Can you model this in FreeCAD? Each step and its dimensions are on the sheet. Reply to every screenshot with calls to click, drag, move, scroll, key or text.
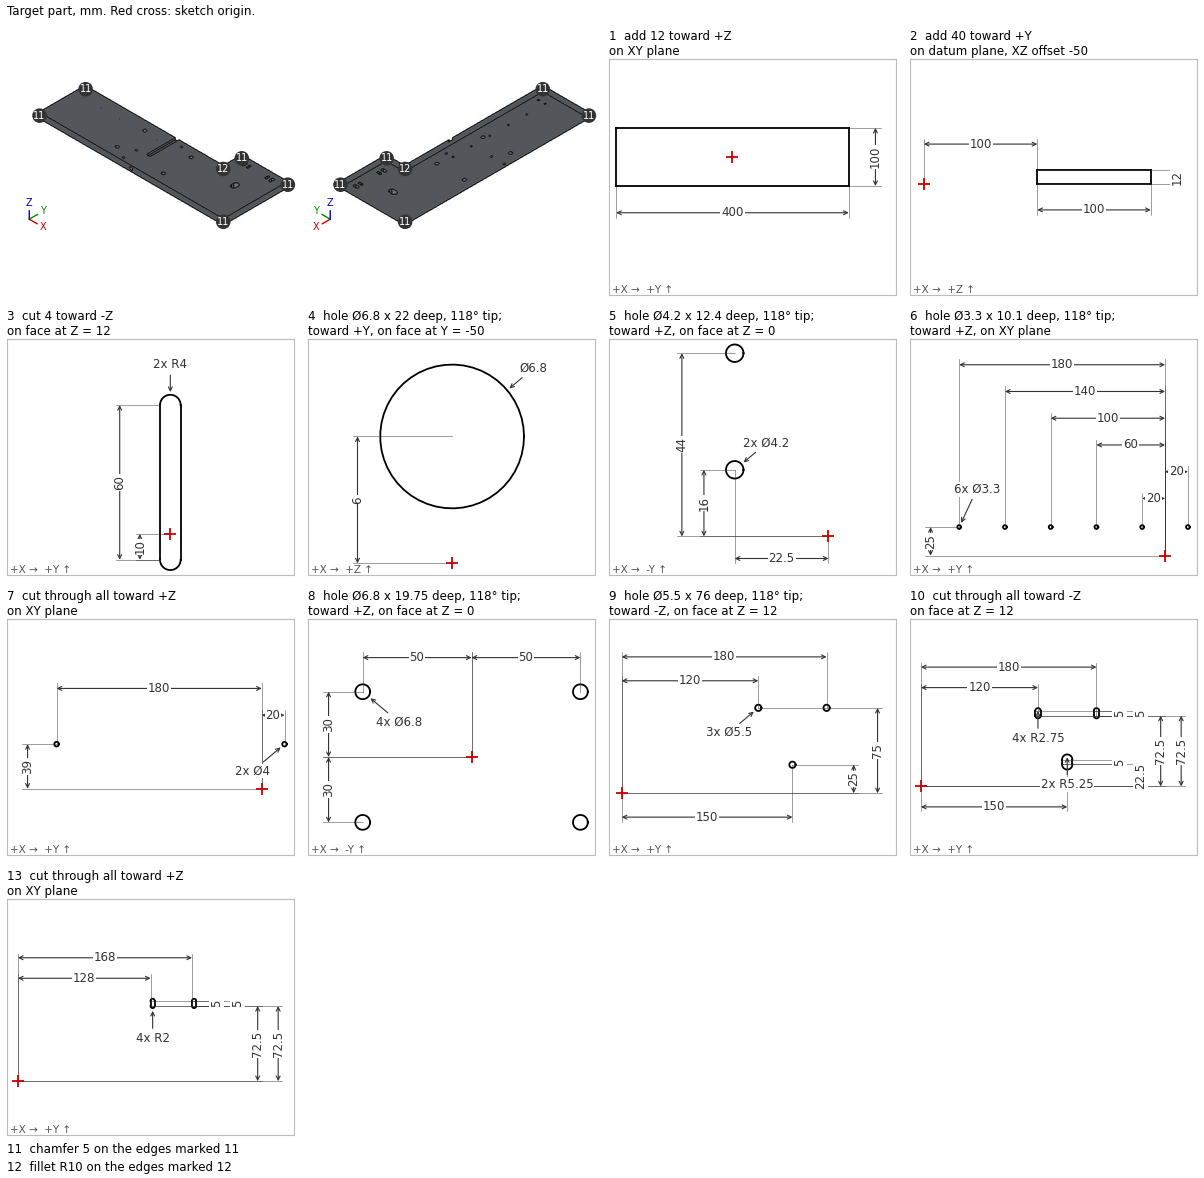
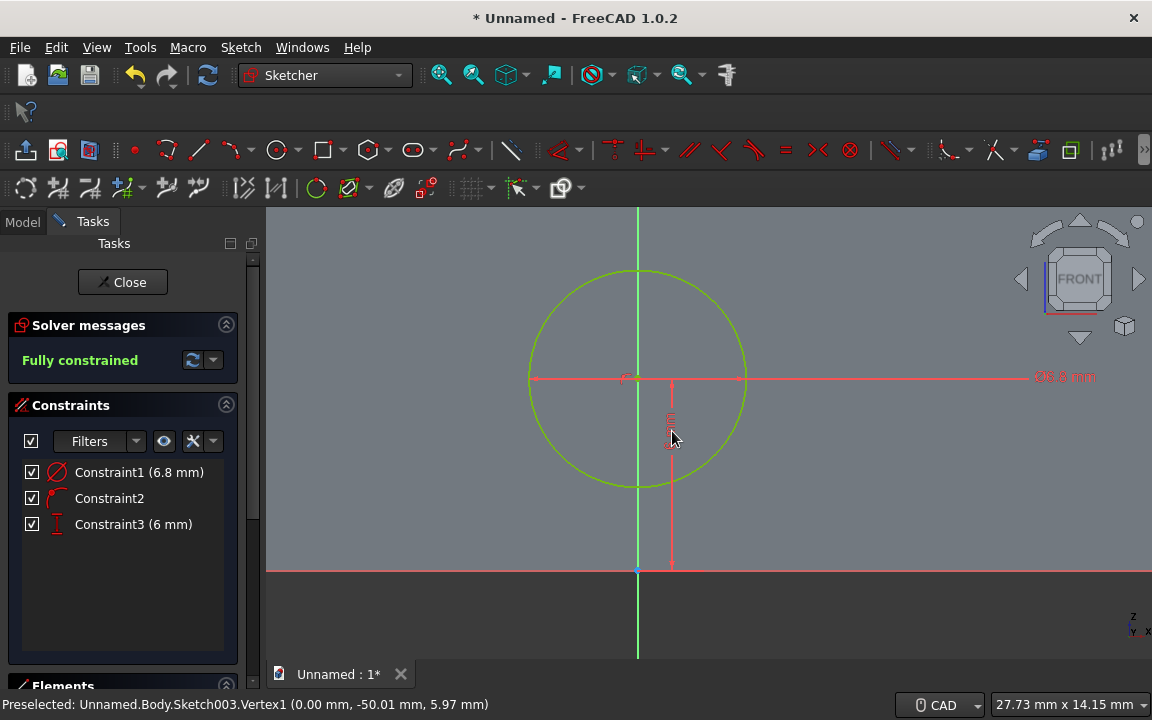
click(123, 282)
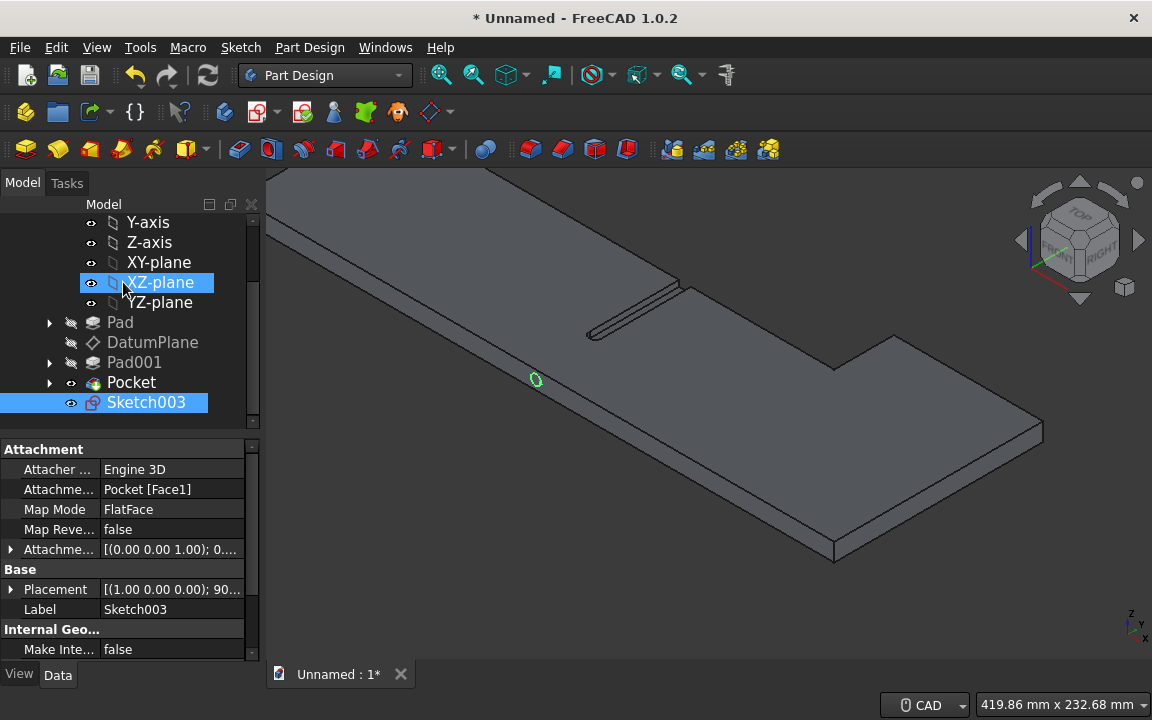
click(272, 150)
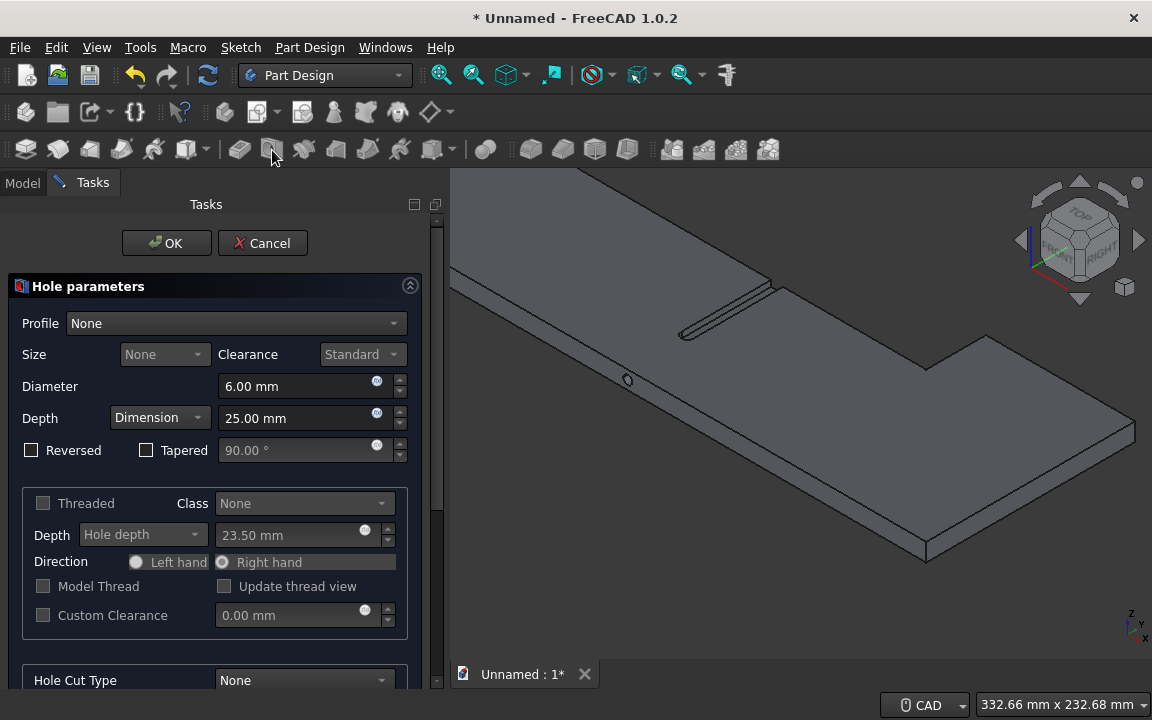
triple_click(305, 386)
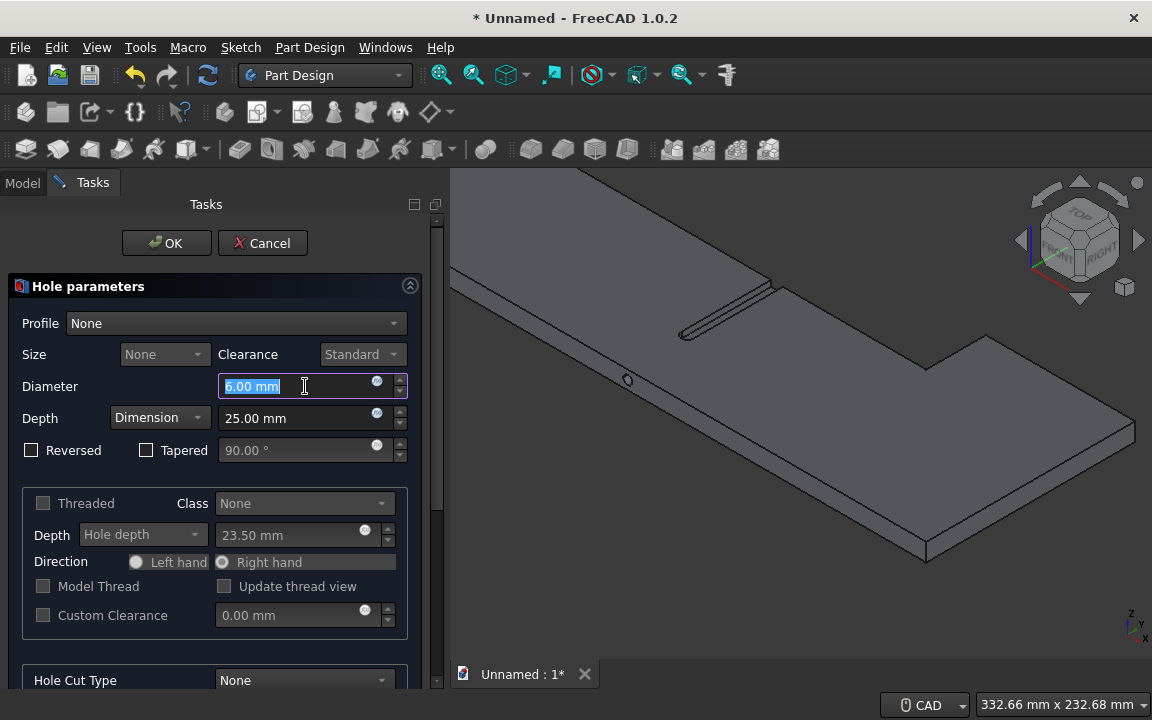
text(6.8)
key(Tab)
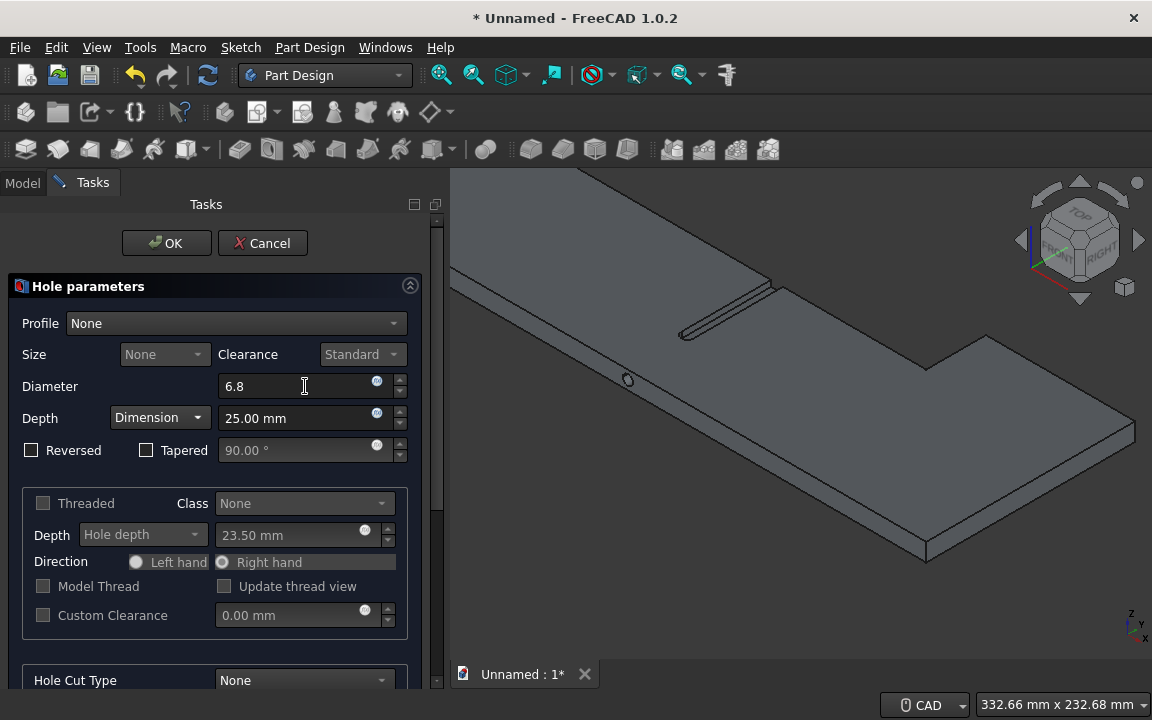
triple_click(305, 418)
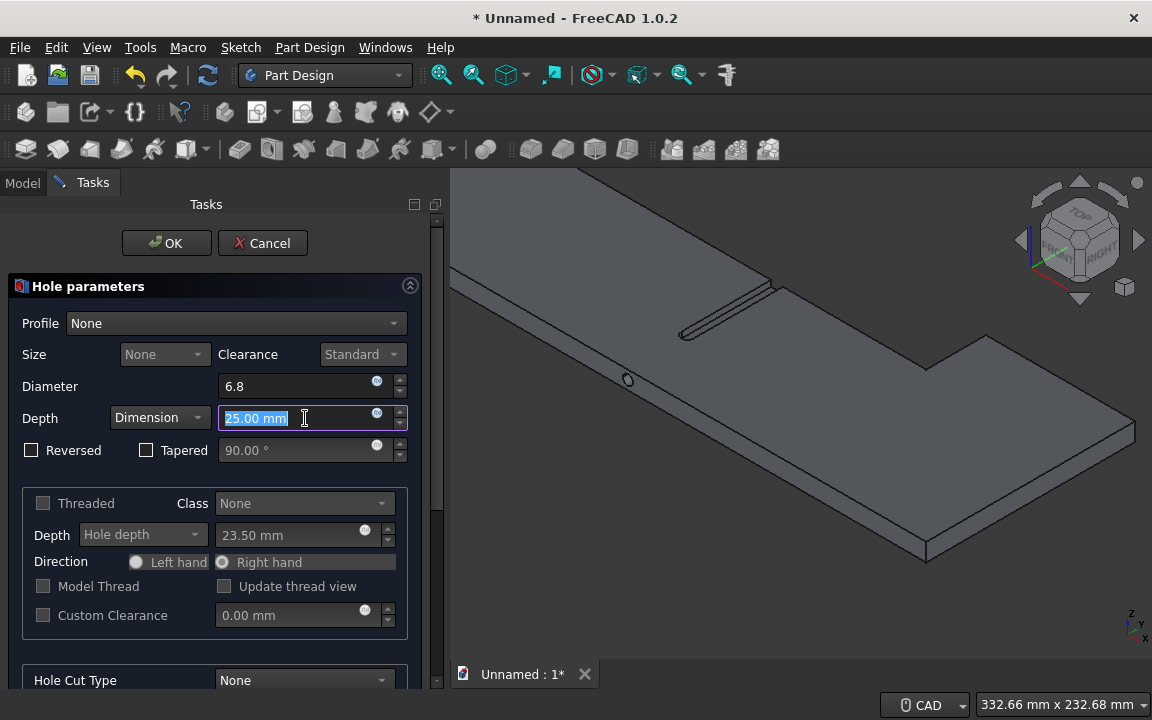
text(22)
key(Tab)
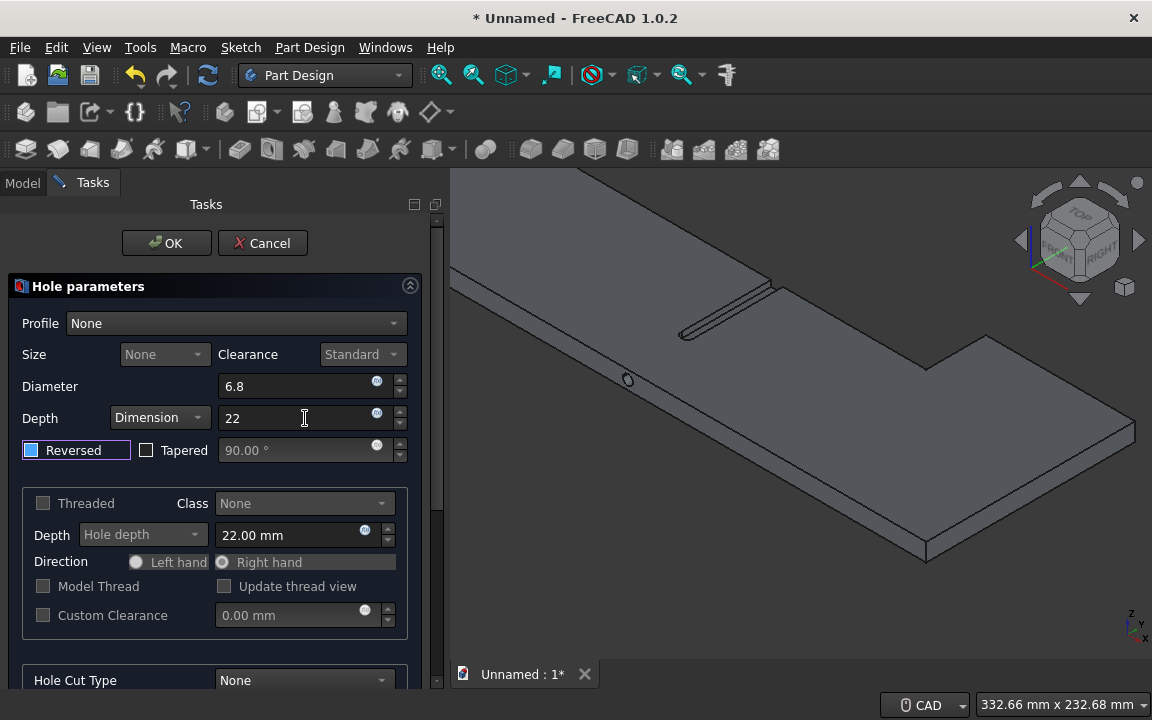
click(167, 243)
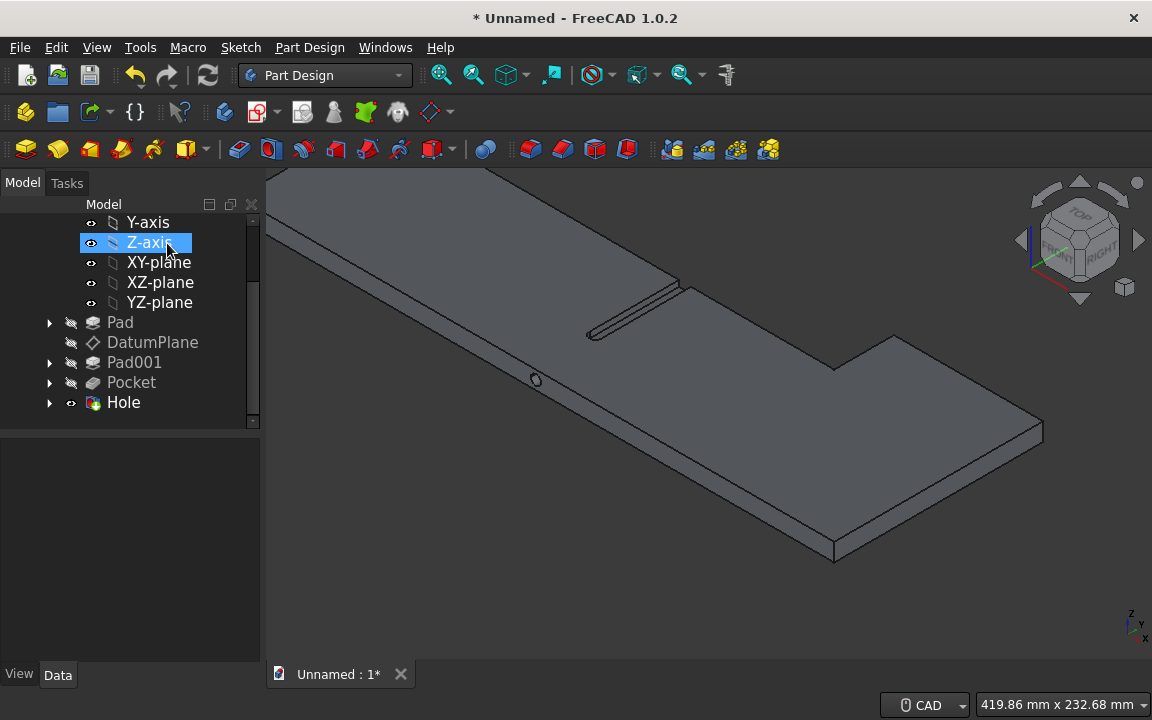
click(442, 76)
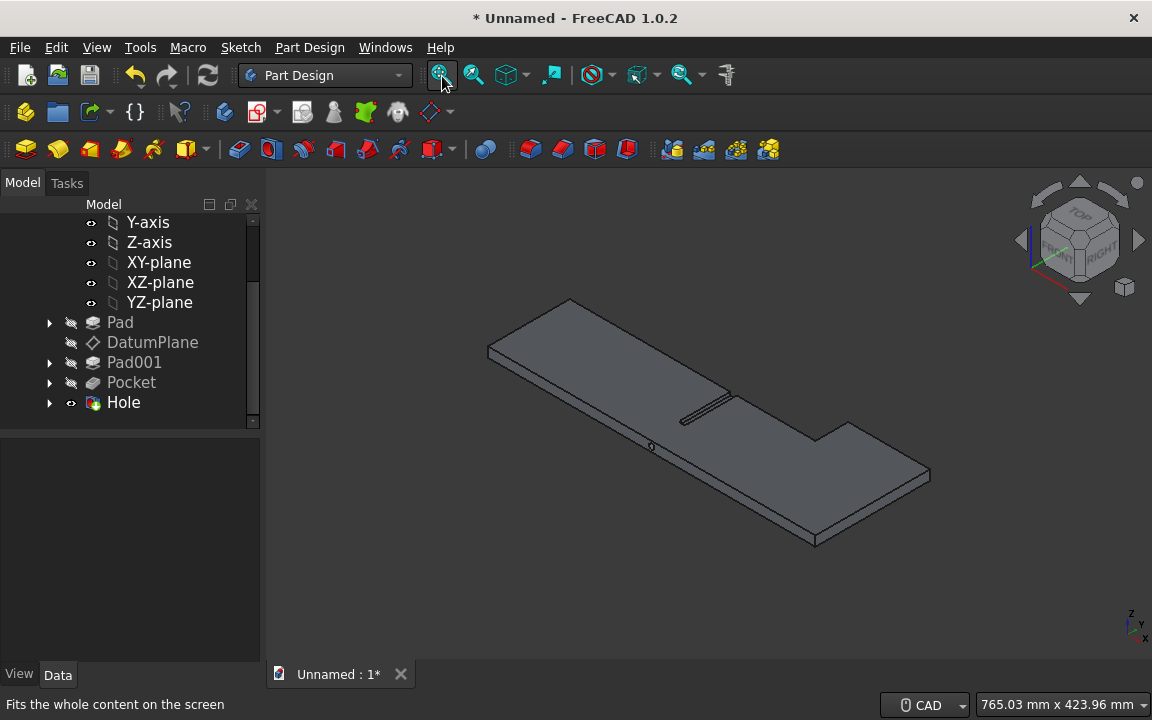
key(5)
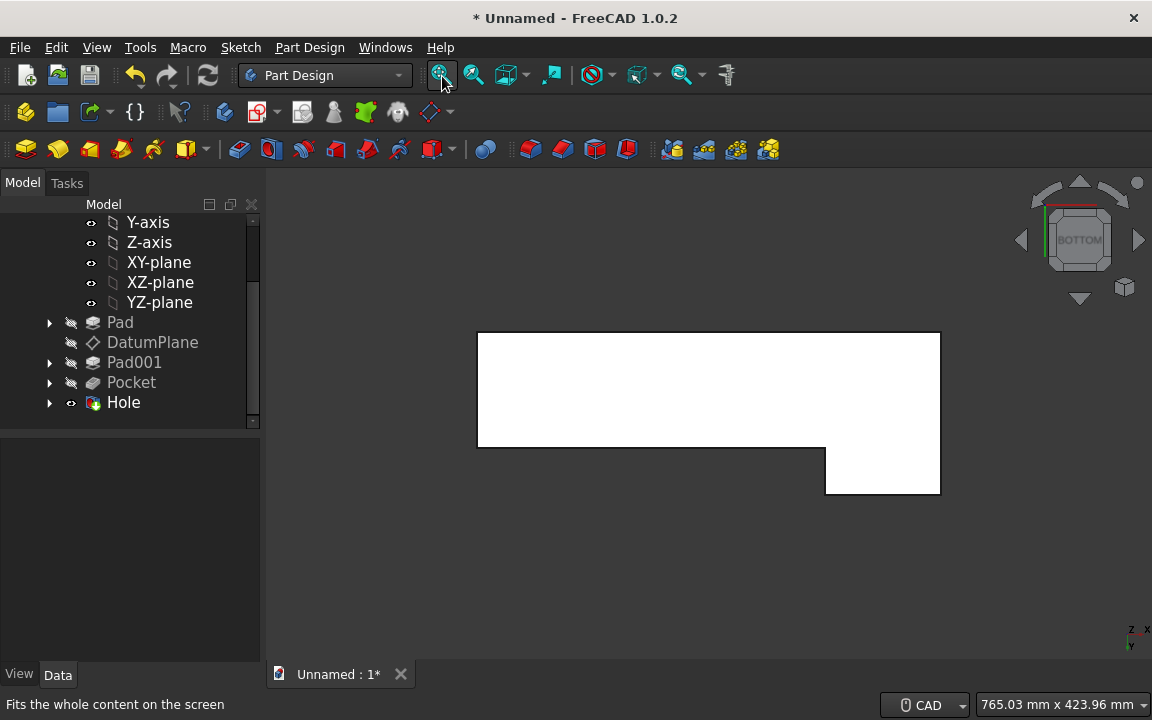
click(841, 389)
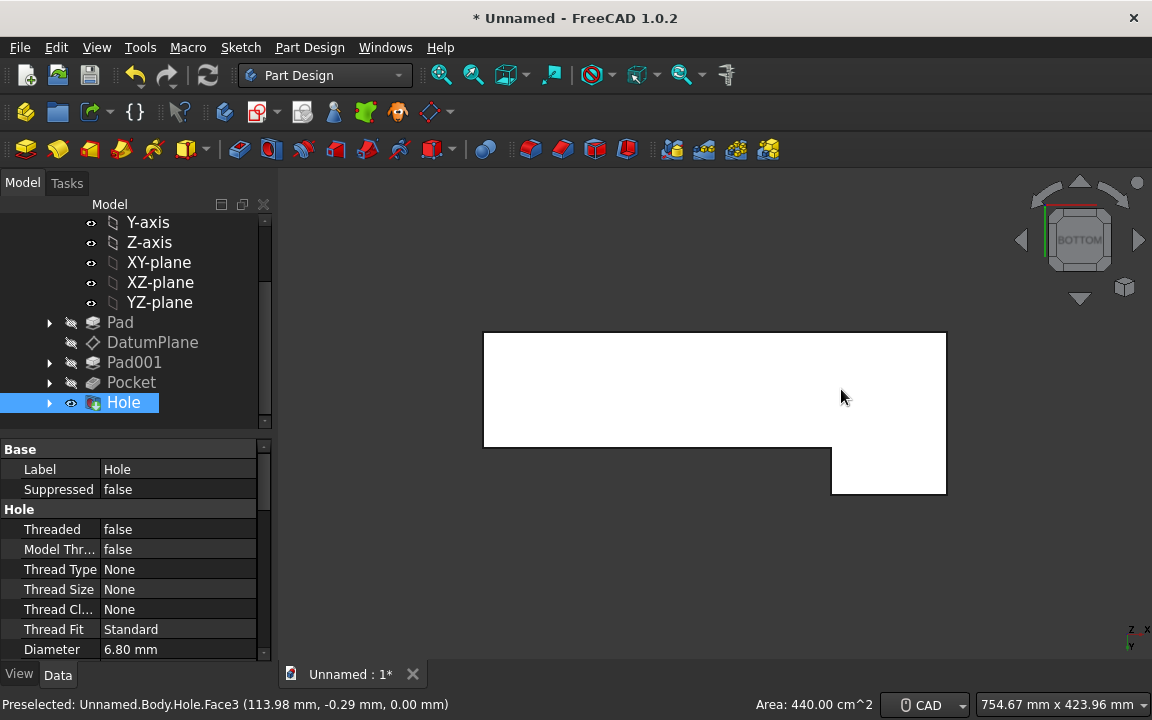
click(258, 112)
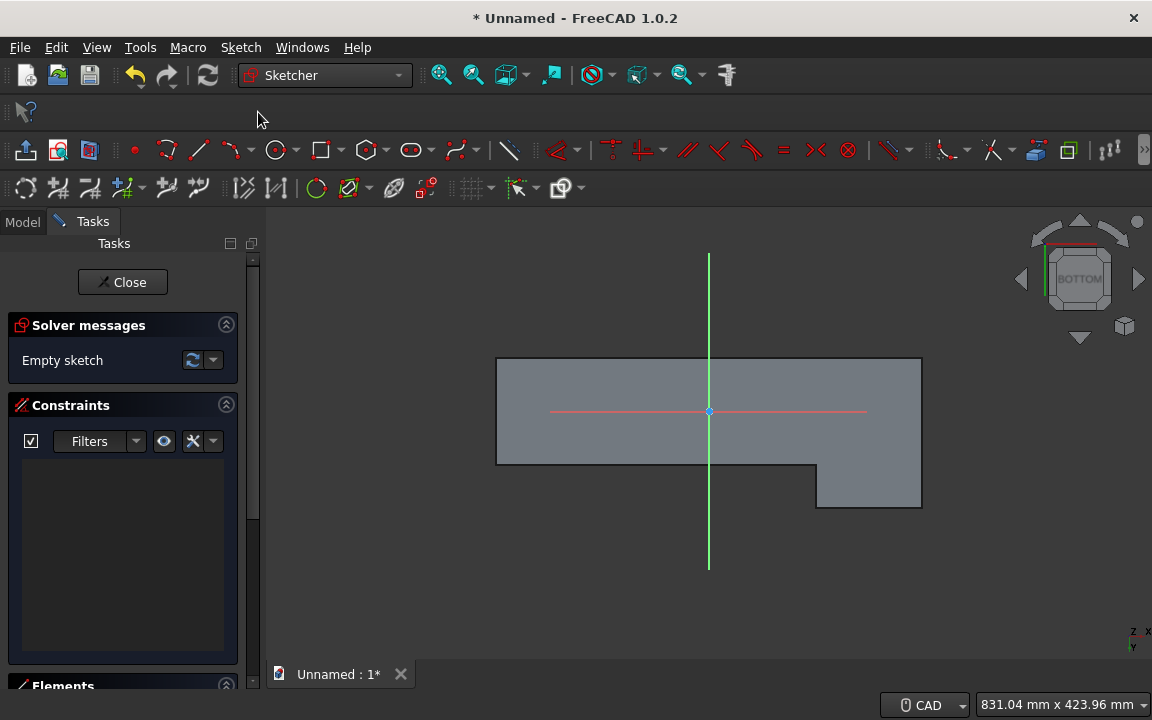
scroll(707, 378, up, 9)